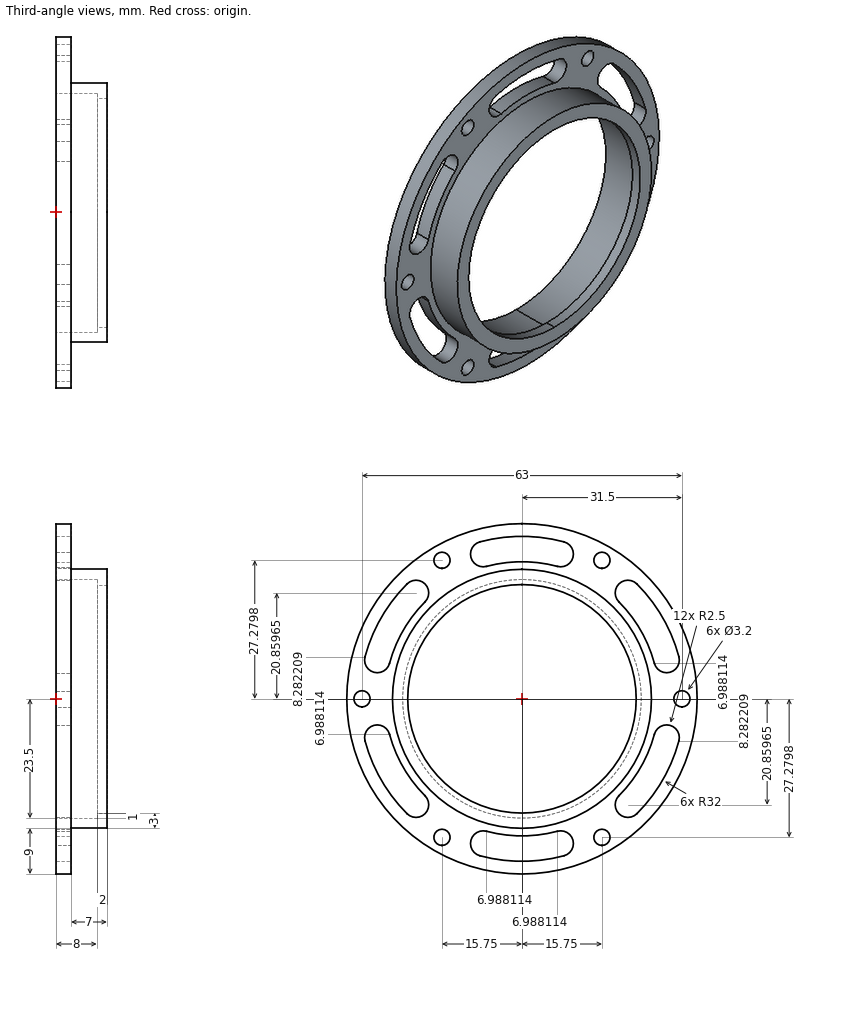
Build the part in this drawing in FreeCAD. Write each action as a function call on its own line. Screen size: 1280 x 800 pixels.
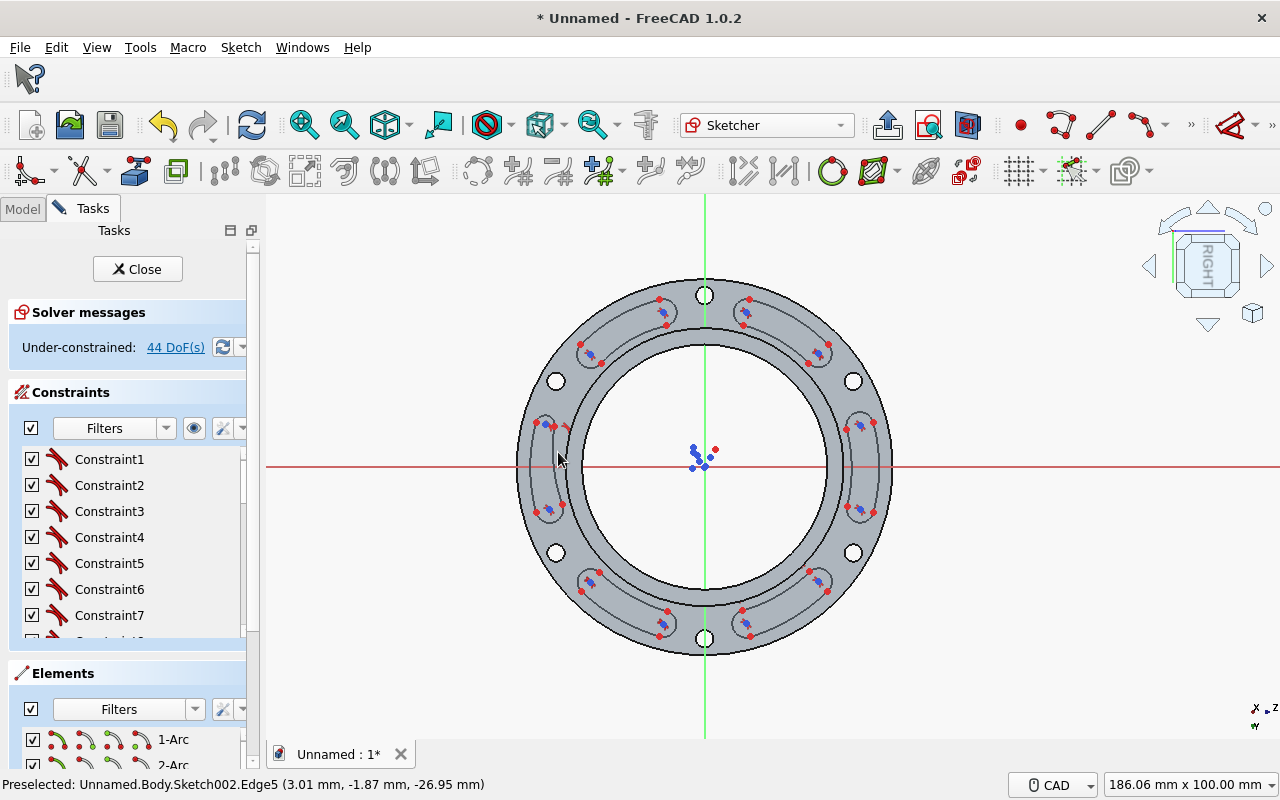
click(603, 609)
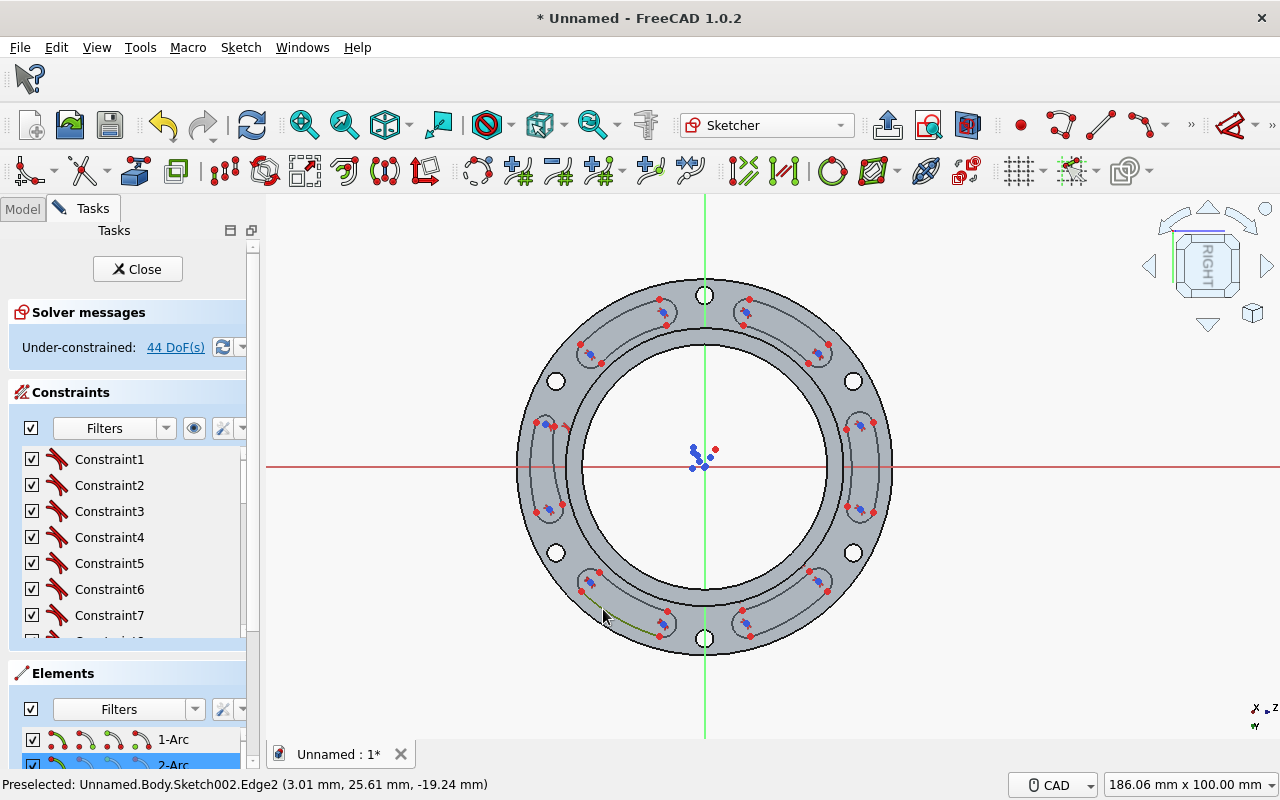
click(531, 449)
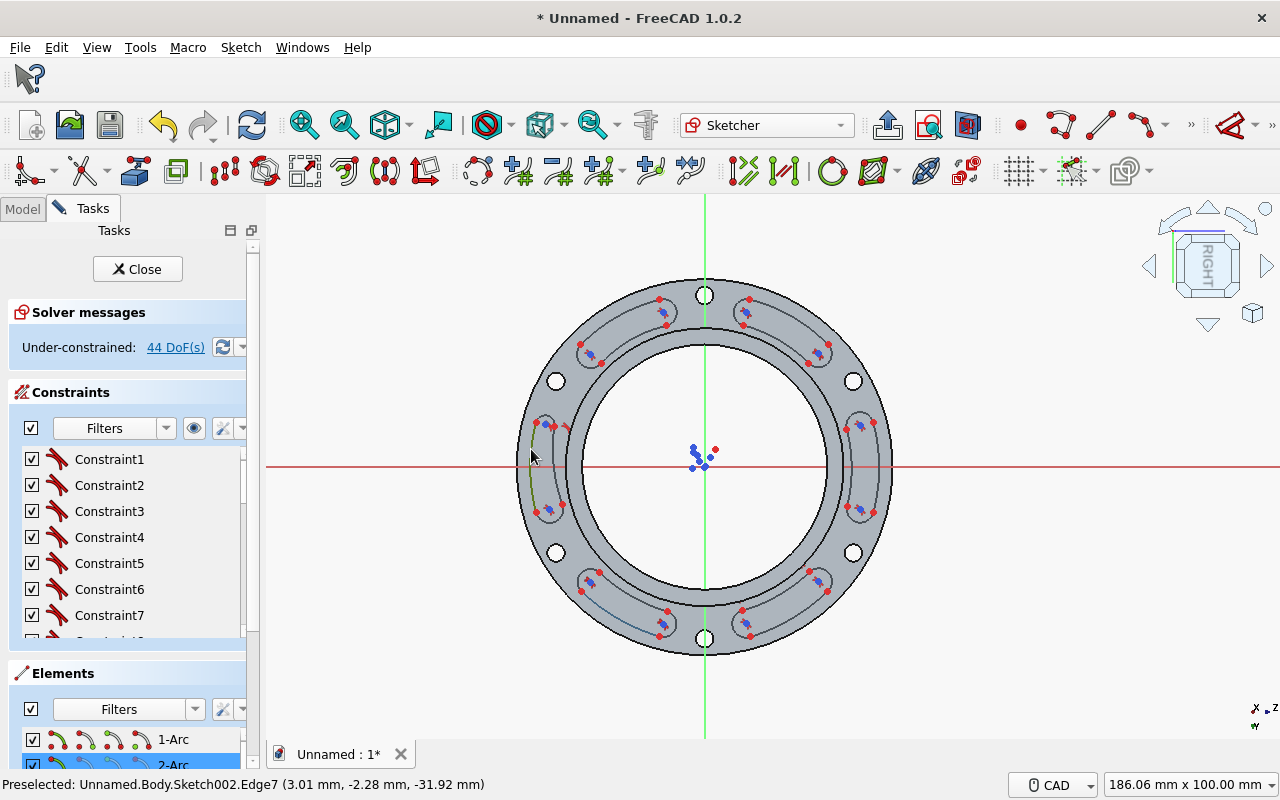
key(c)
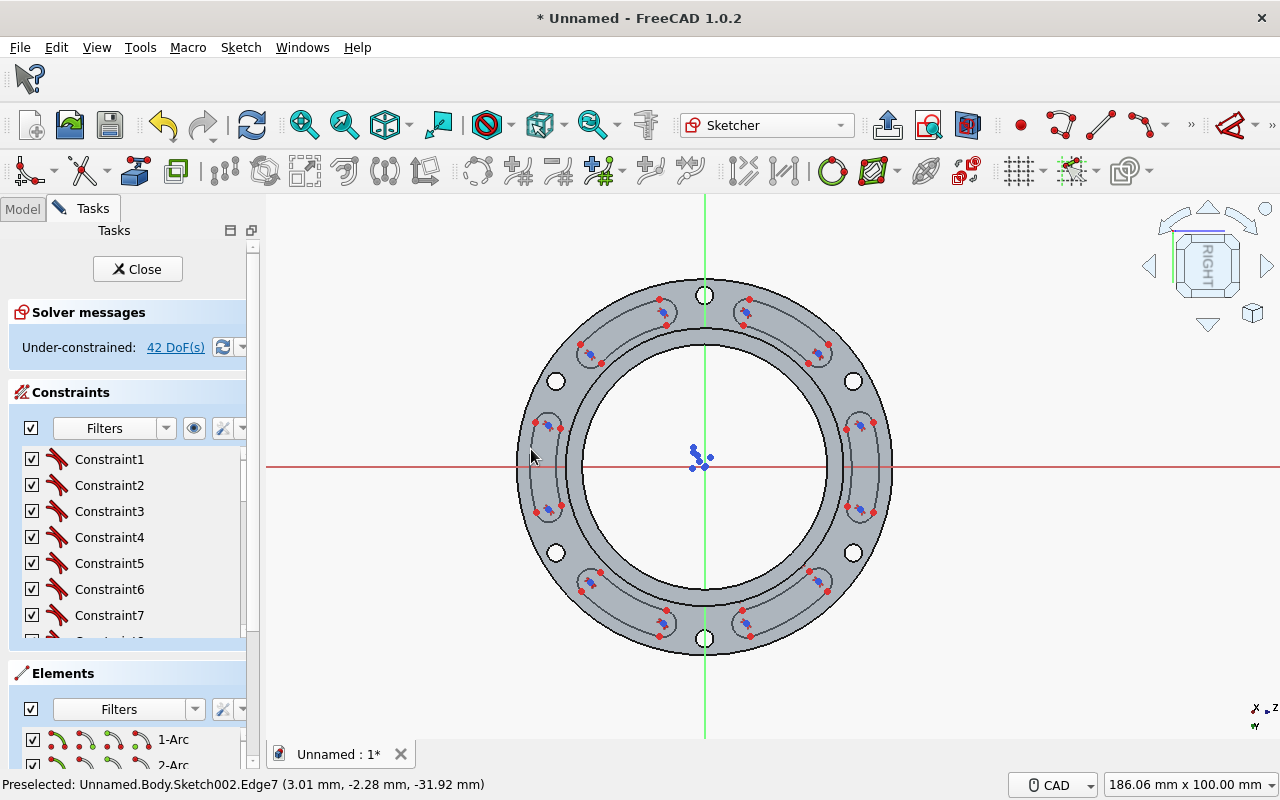
click(602, 609)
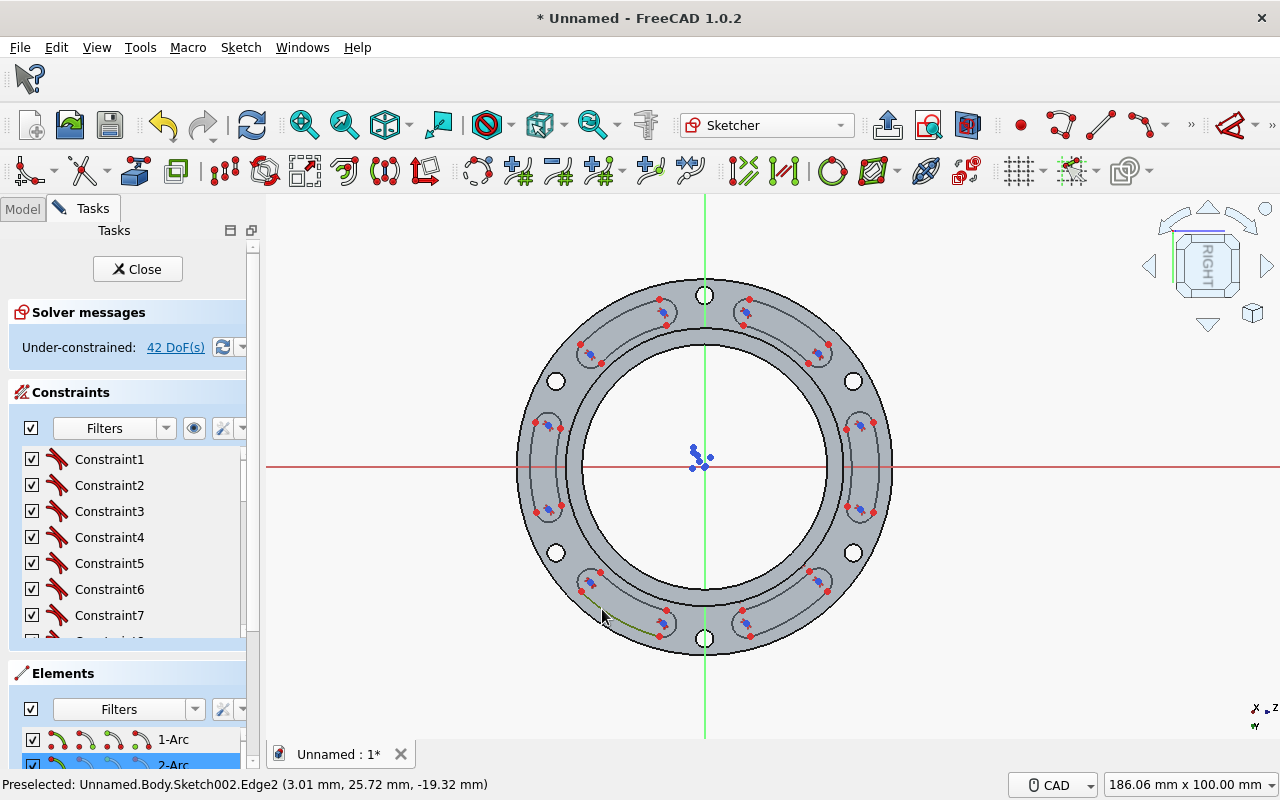
click(644, 333)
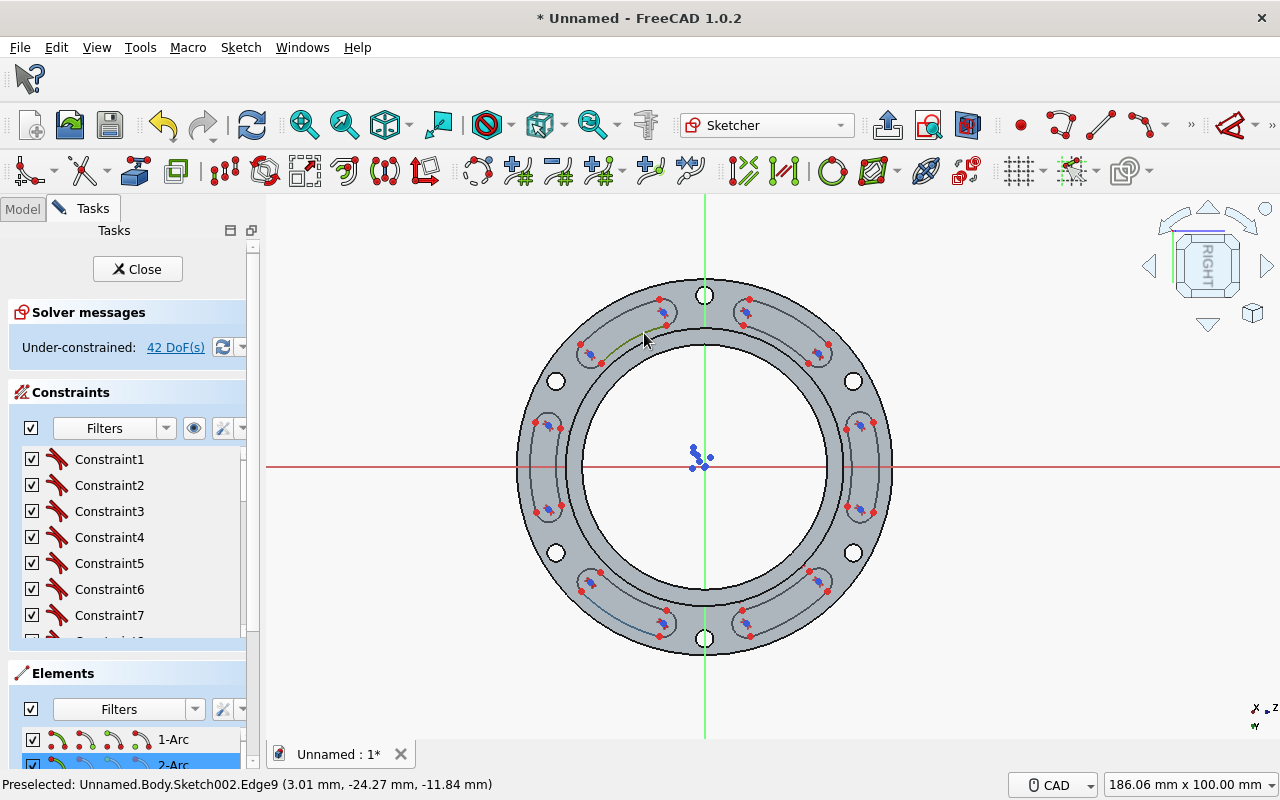
key(c)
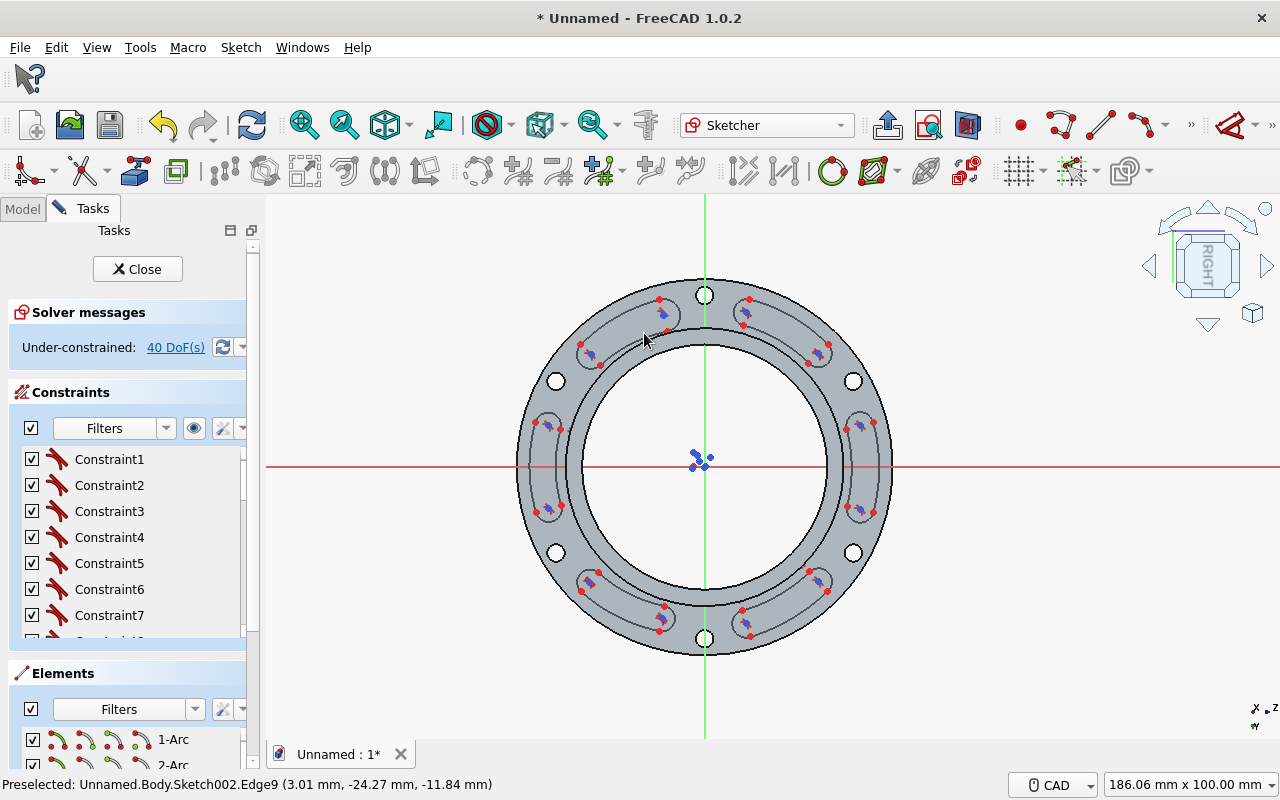
click(603, 608)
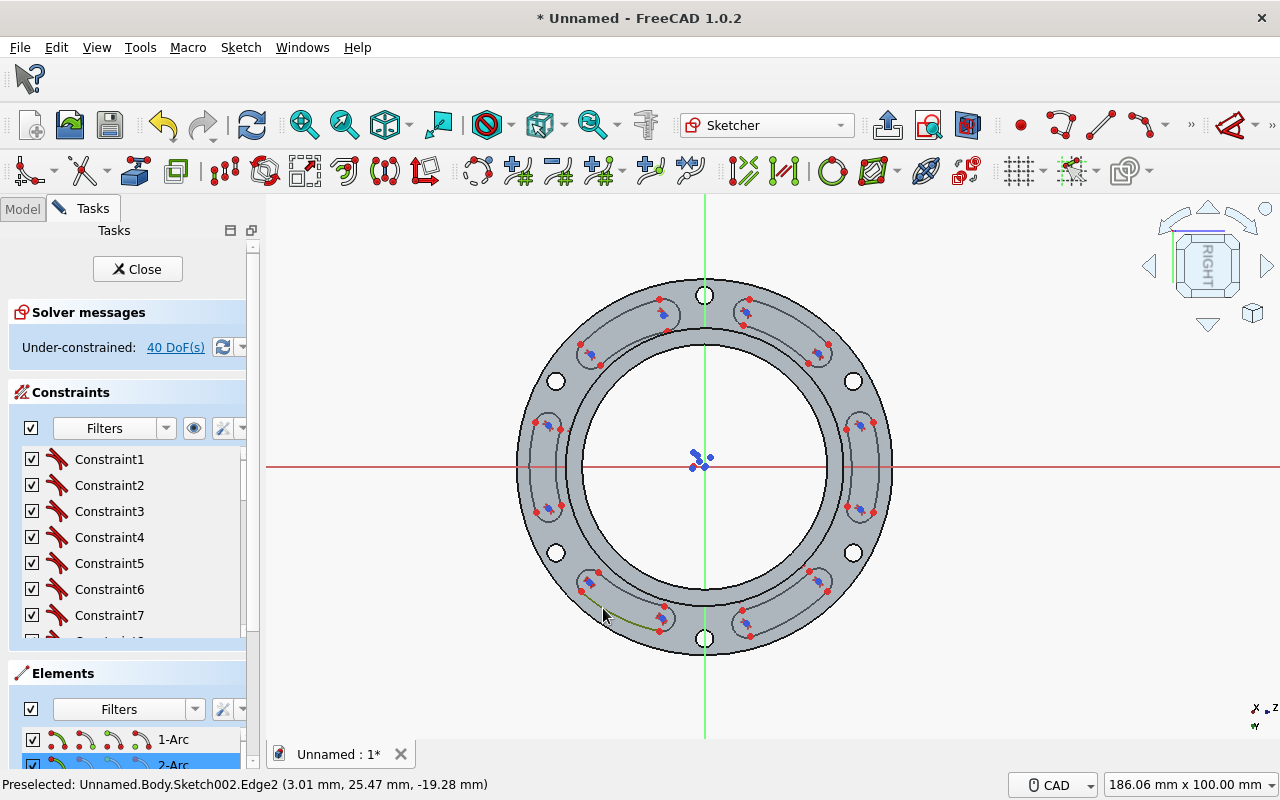
click(634, 308)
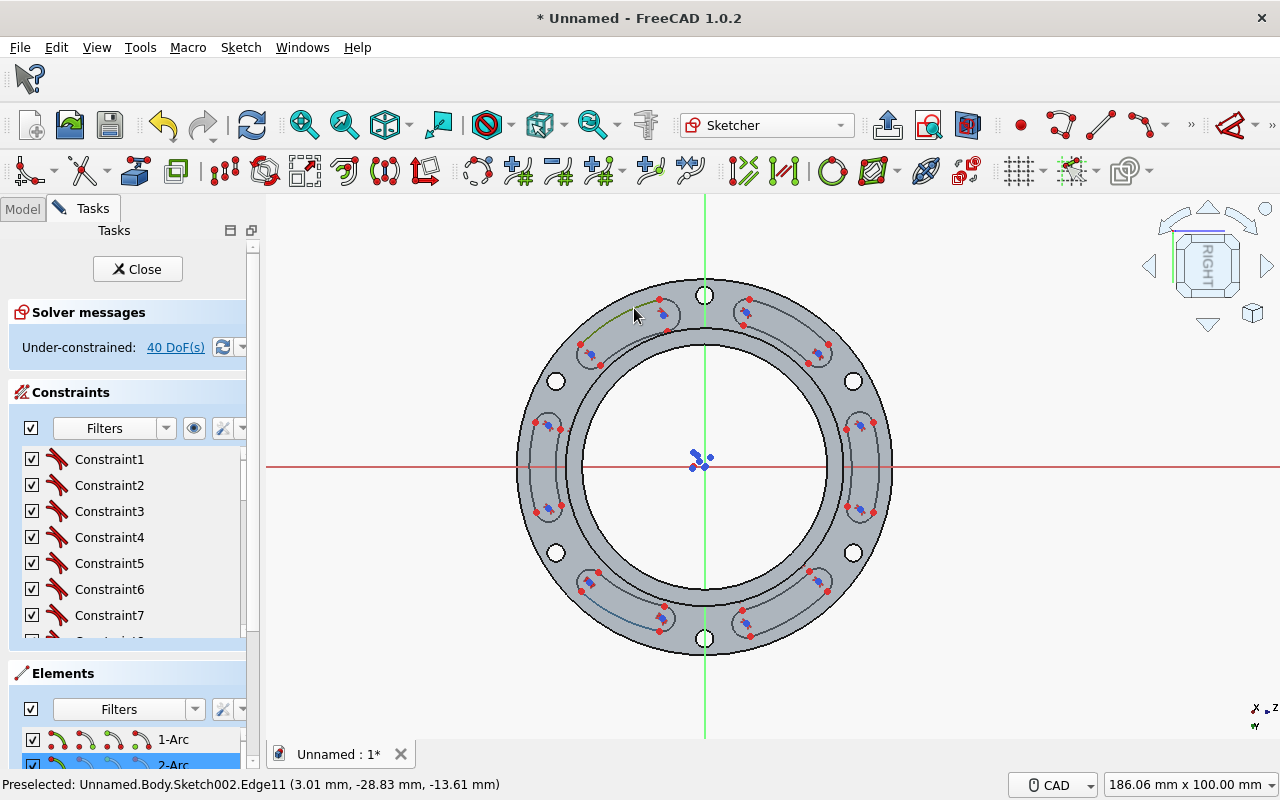
key(c)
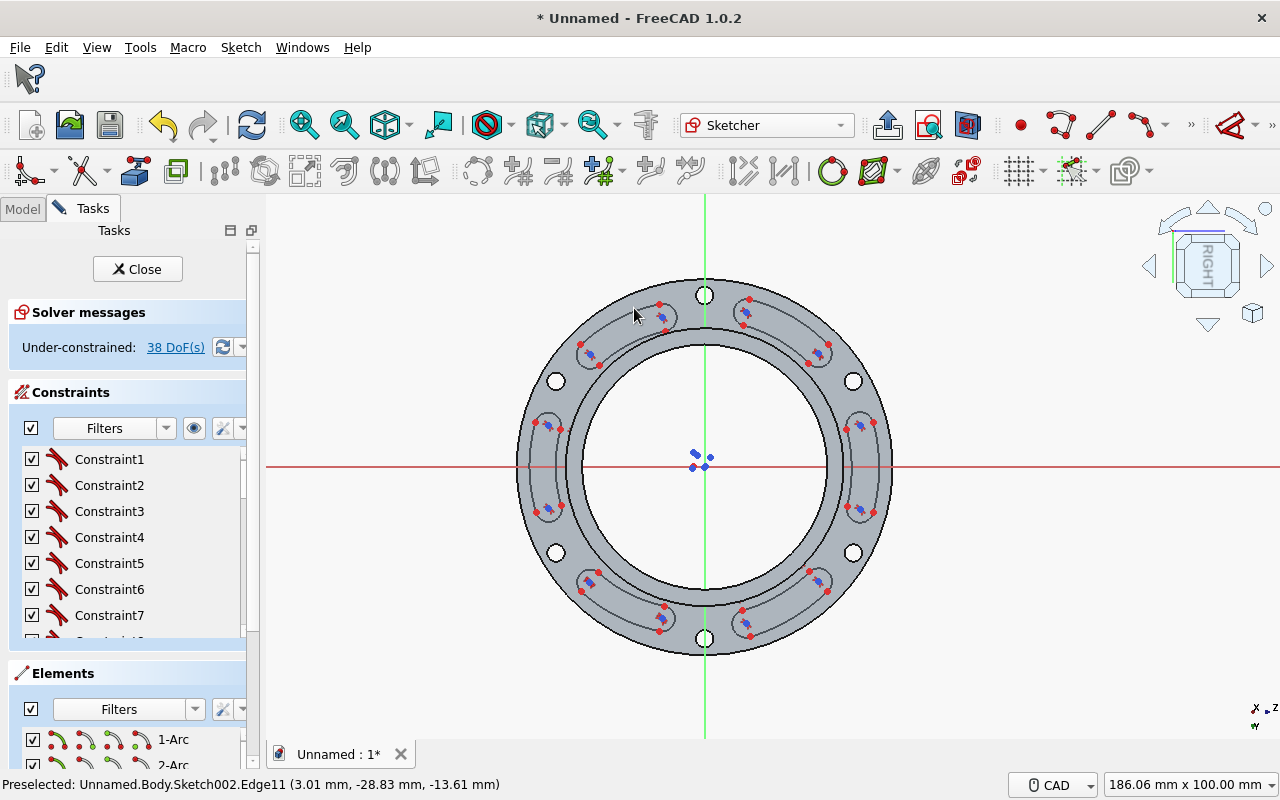
click(603, 608)